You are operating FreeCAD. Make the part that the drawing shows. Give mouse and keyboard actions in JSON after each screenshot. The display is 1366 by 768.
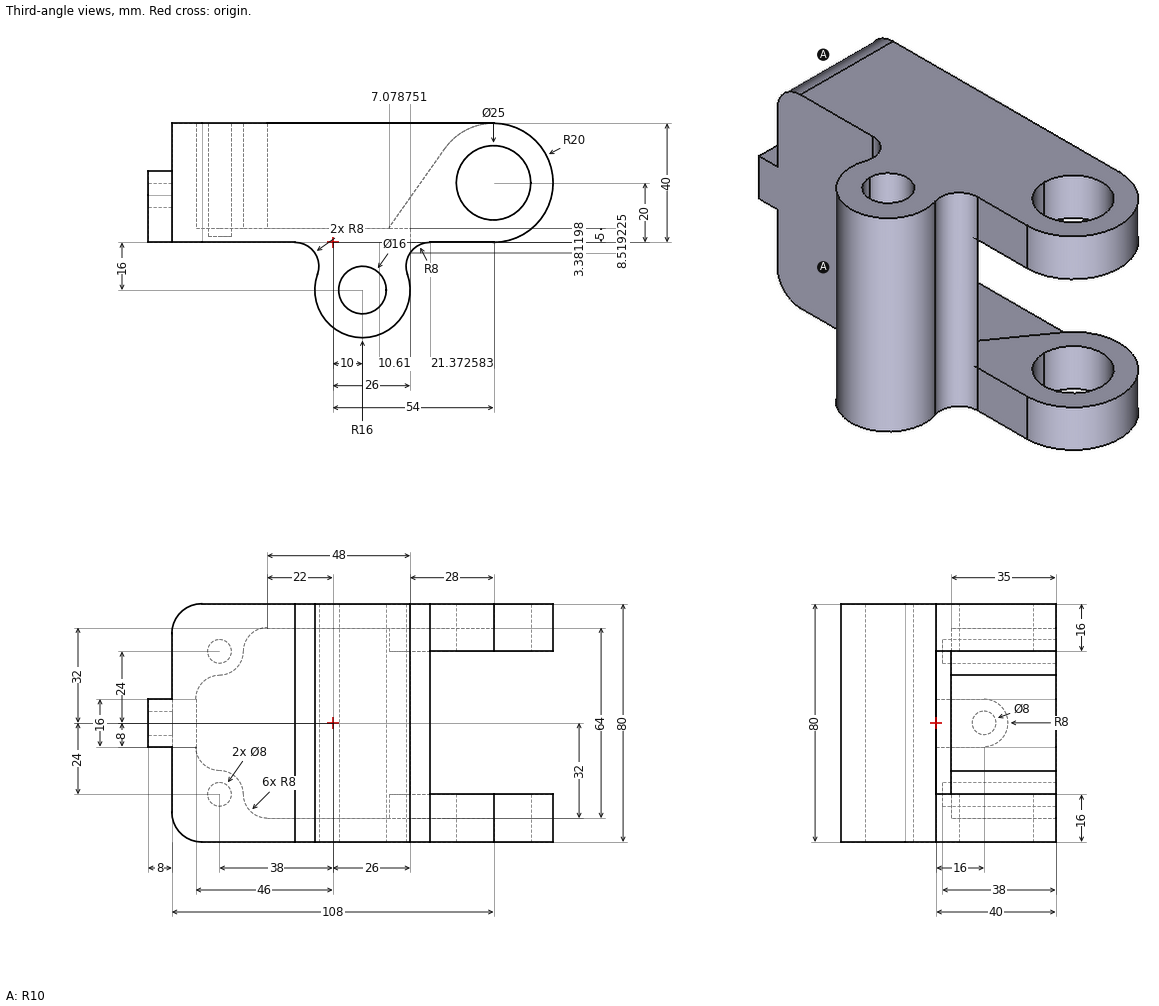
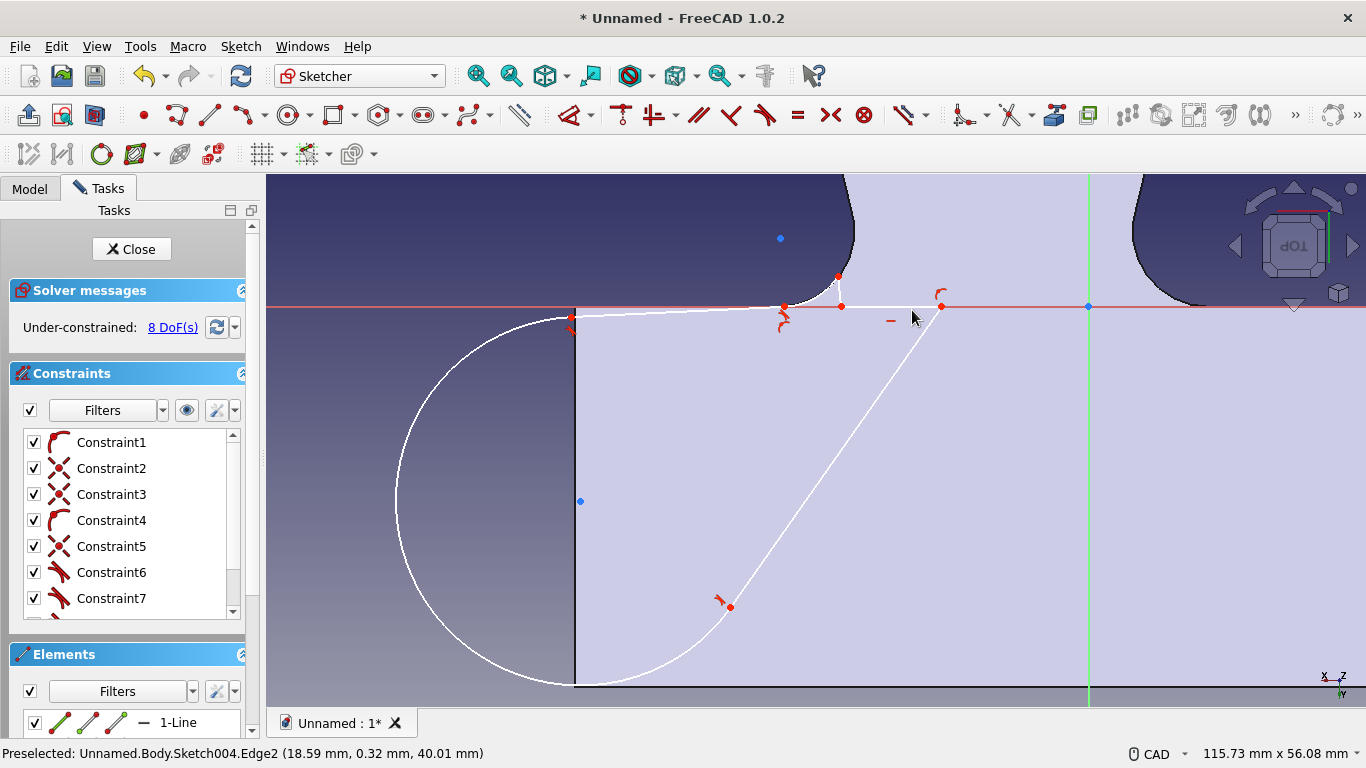
{"action": "left_click", "coordinate": [720, 310]}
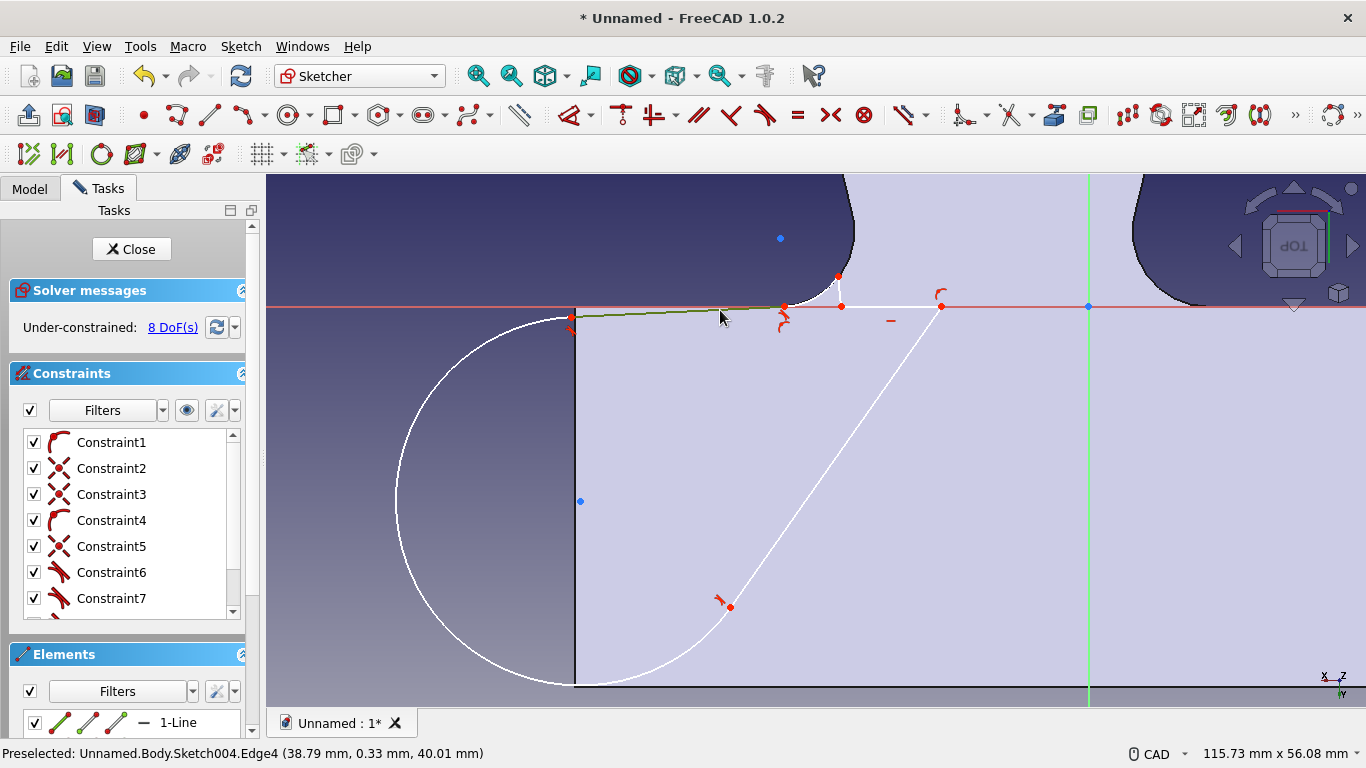
{"action": "left_click", "coordinate": [676, 116]}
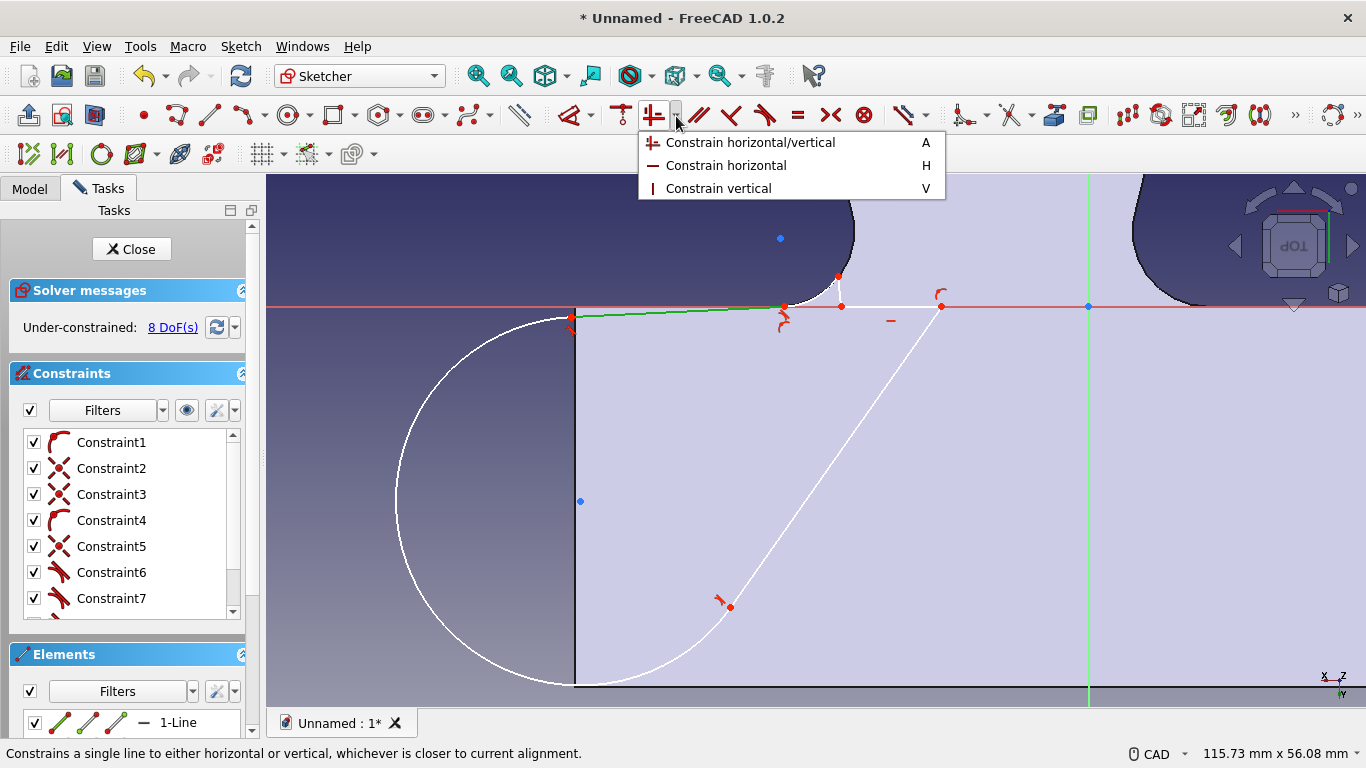
{"action": "left_click", "coordinate": [792, 166]}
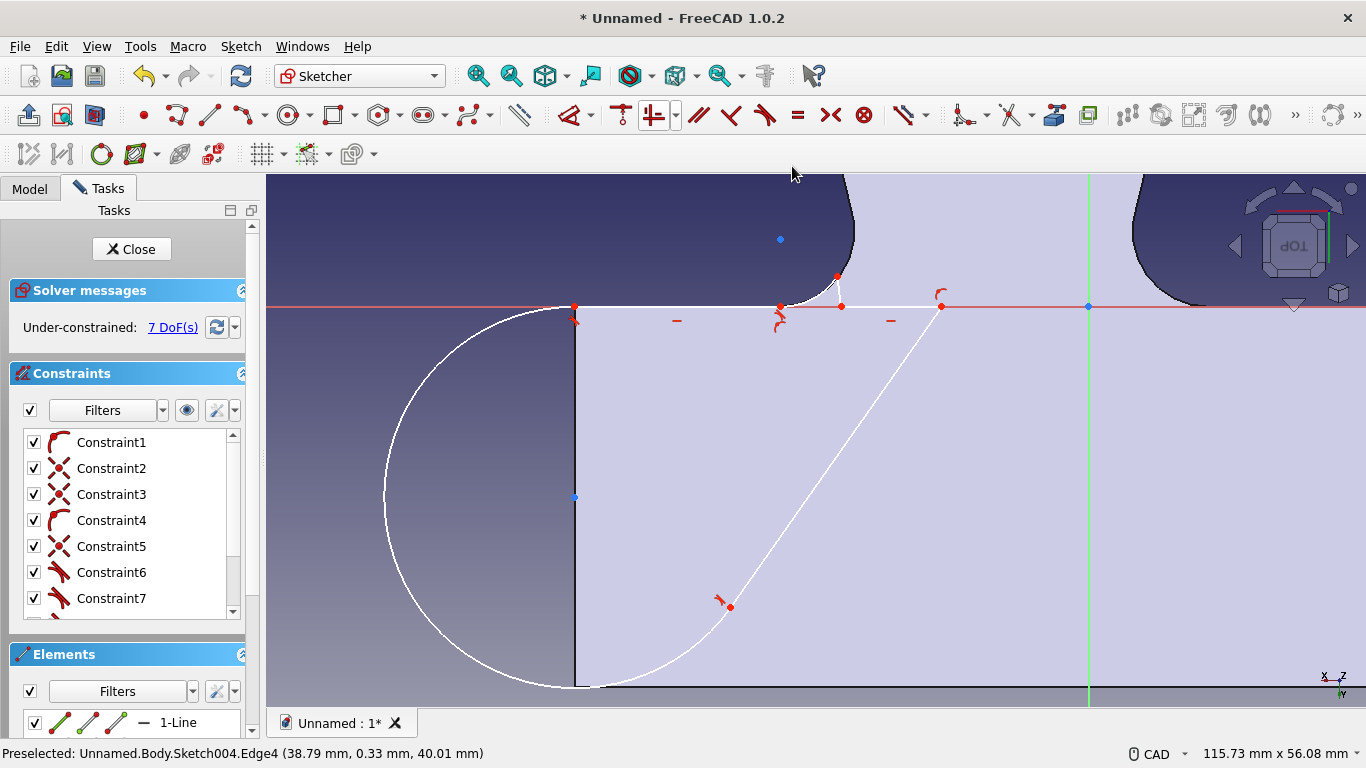
{"action": "left_click", "coordinate": [568, 116]}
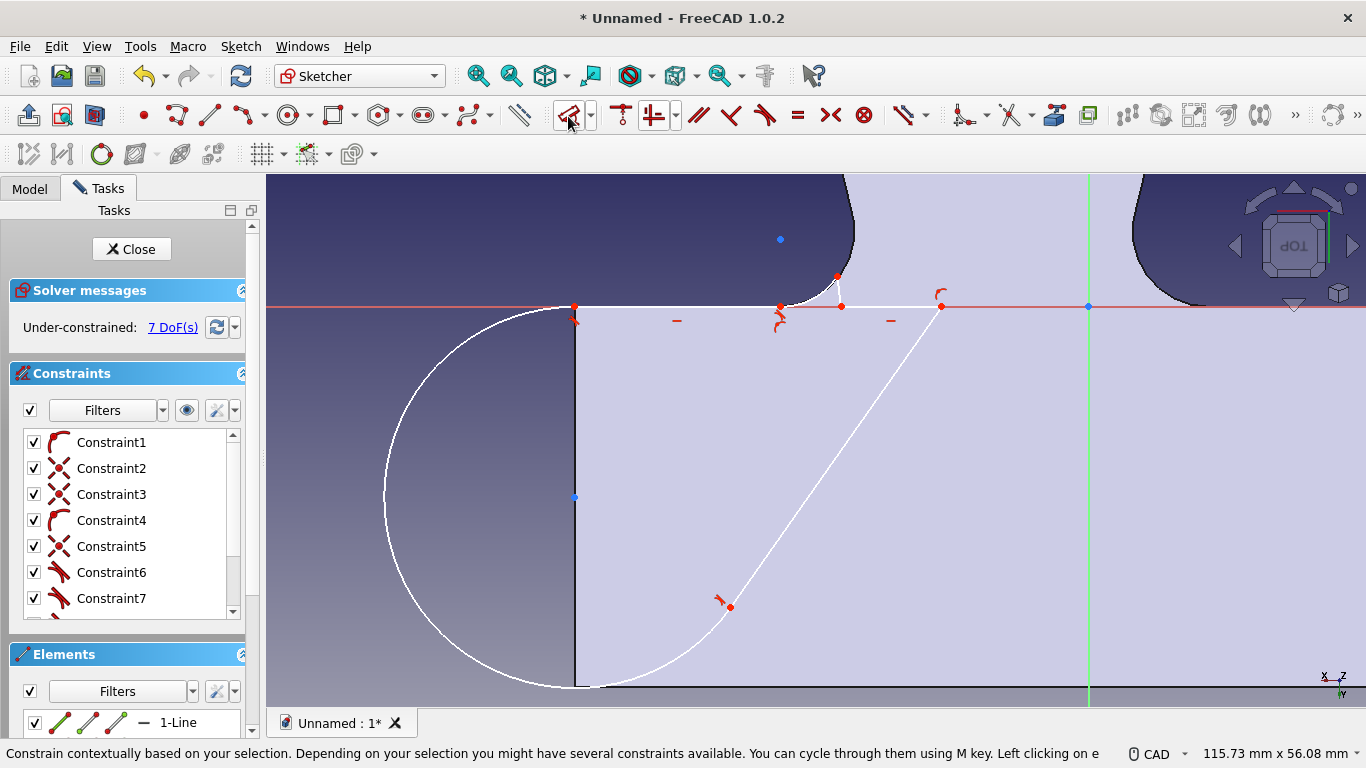
{"action": "left_click", "coordinate": [801, 304]}
{"action": "left_click", "coordinate": [811, 335]}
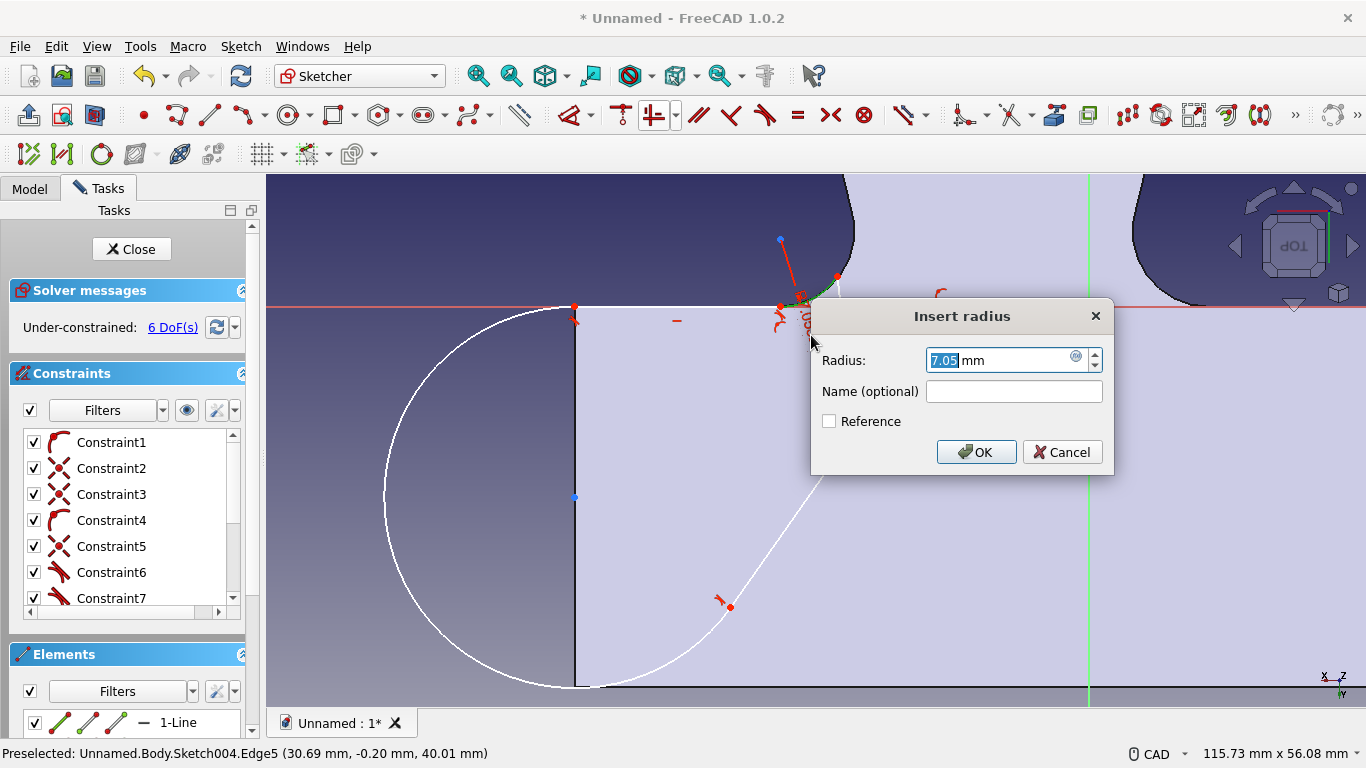
{"action": "type", "text": "8"}
{"action": "key", "text": "Return"}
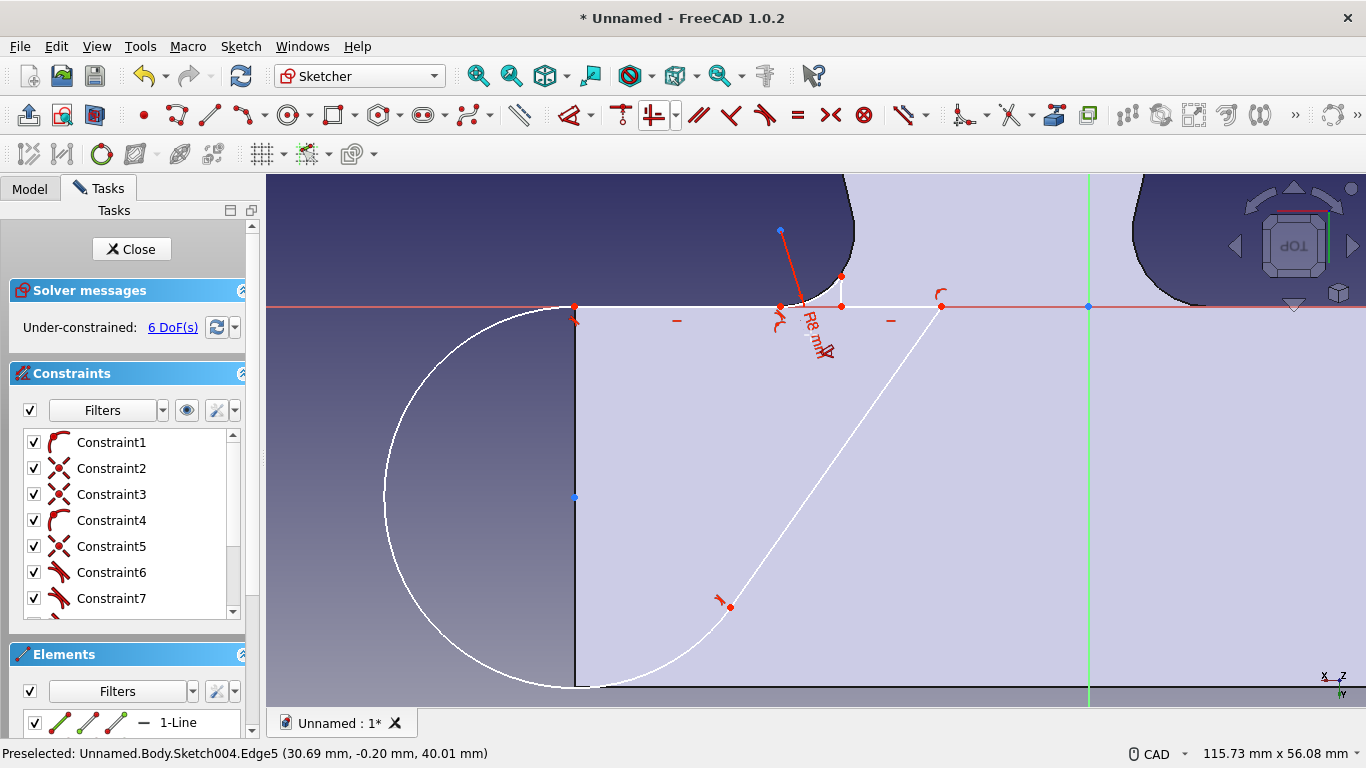
{"action": "left_click", "coordinate": [395, 434]}
{"action": "left_click", "coordinate": [365, 423]}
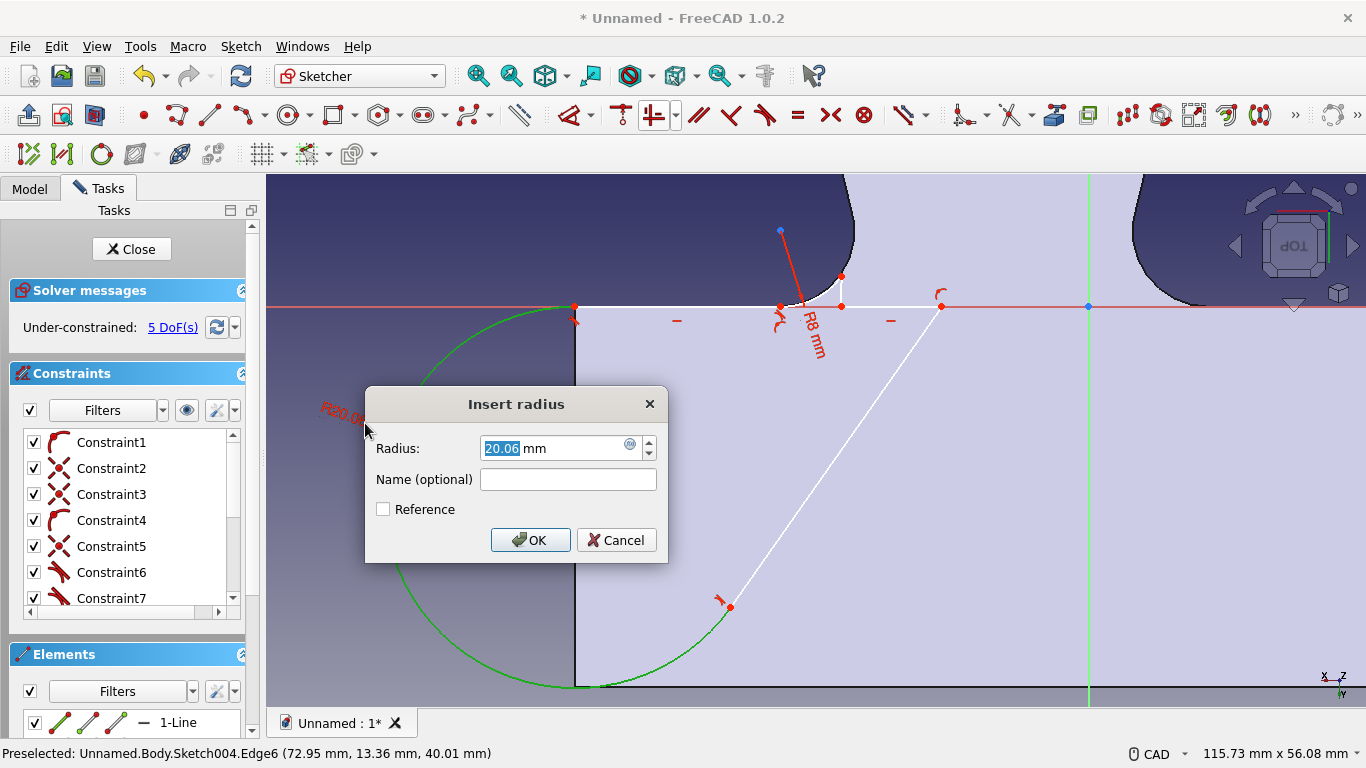
{"action": "type", "text": "20"}
{"action": "key", "text": "Return"}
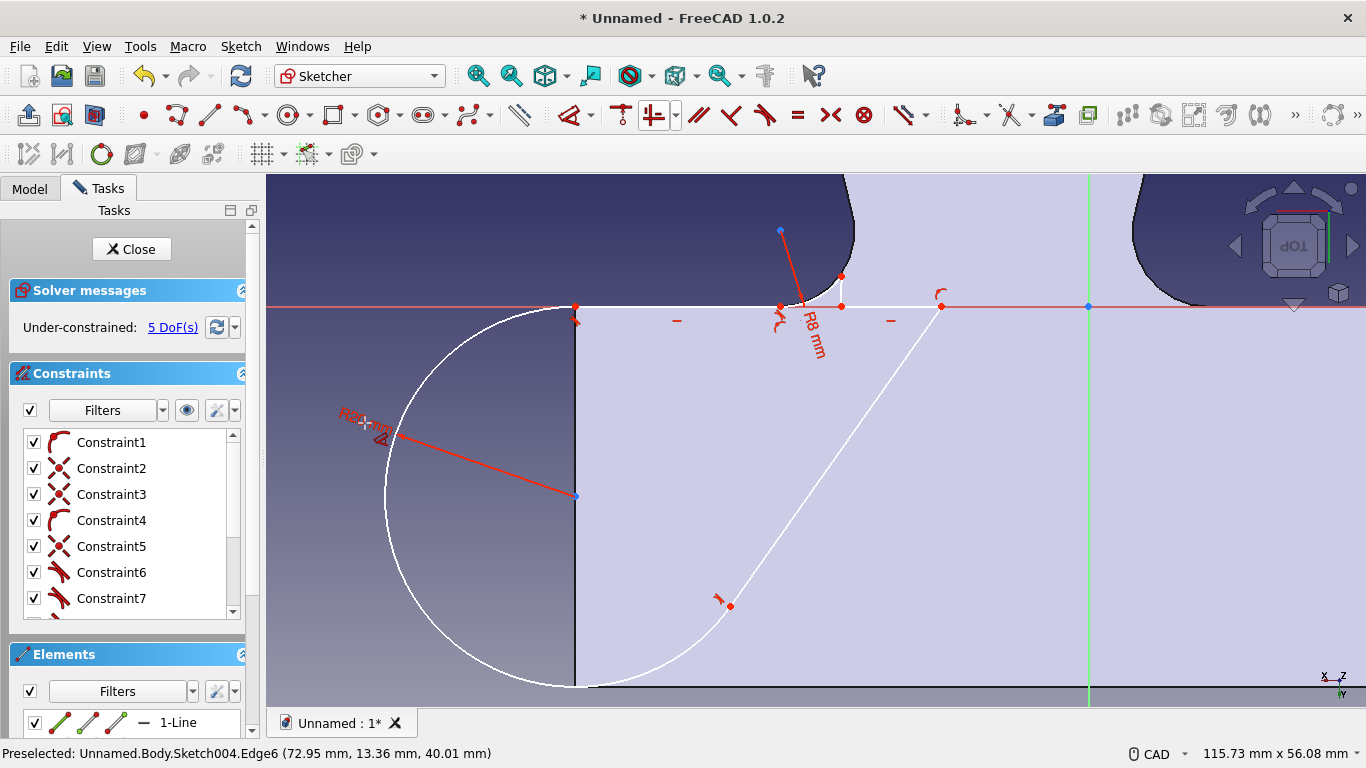
{"action": "left_click", "coordinate": [841, 307]}
{"action": "left_click", "coordinate": [965, 273]}